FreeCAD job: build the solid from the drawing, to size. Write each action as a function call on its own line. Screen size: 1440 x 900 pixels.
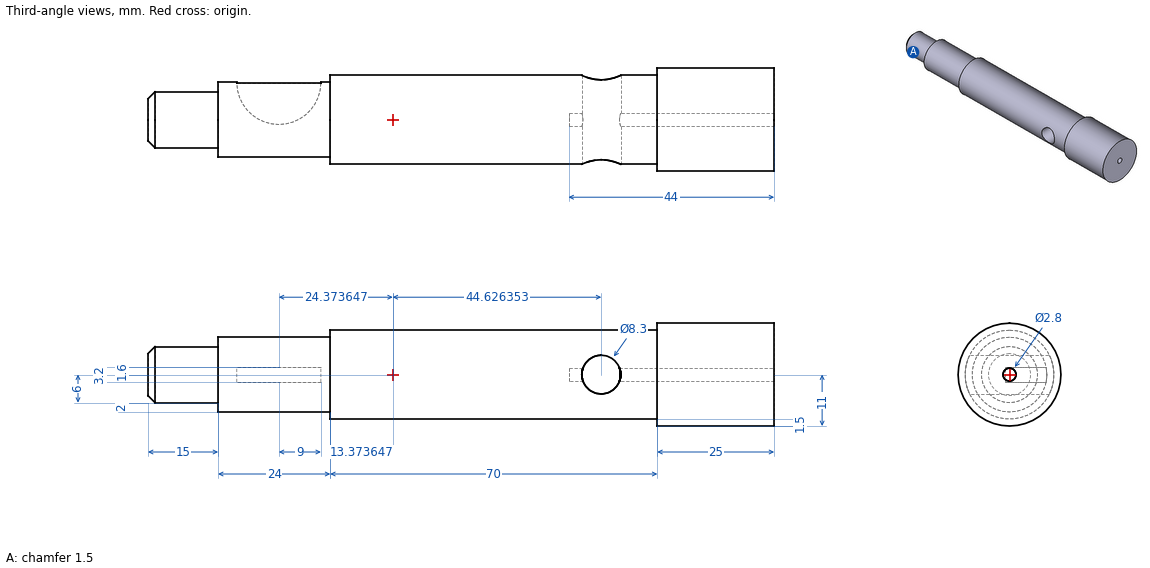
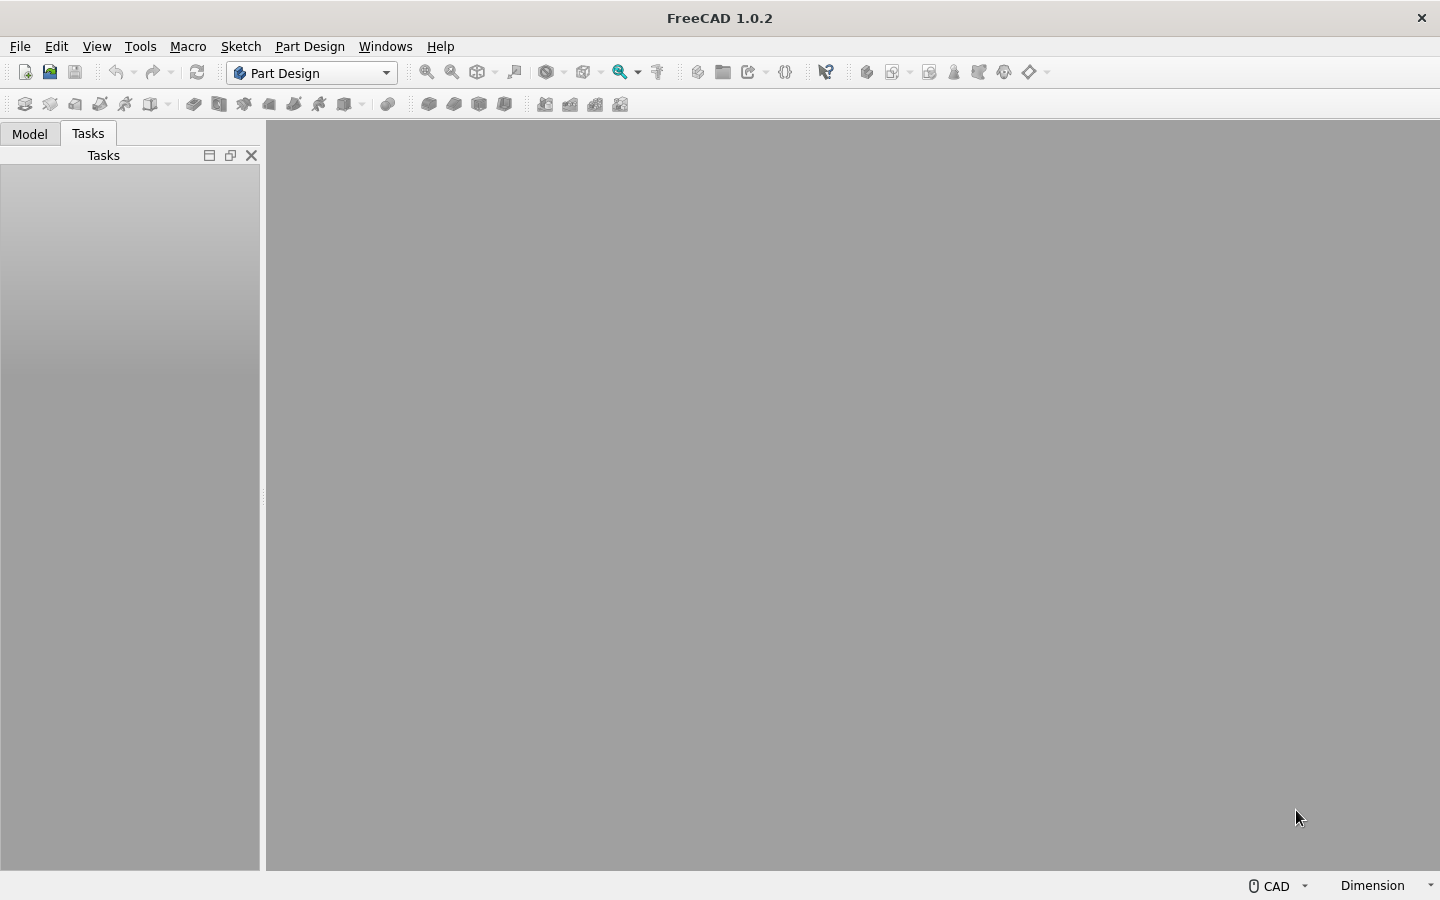
click(25, 72)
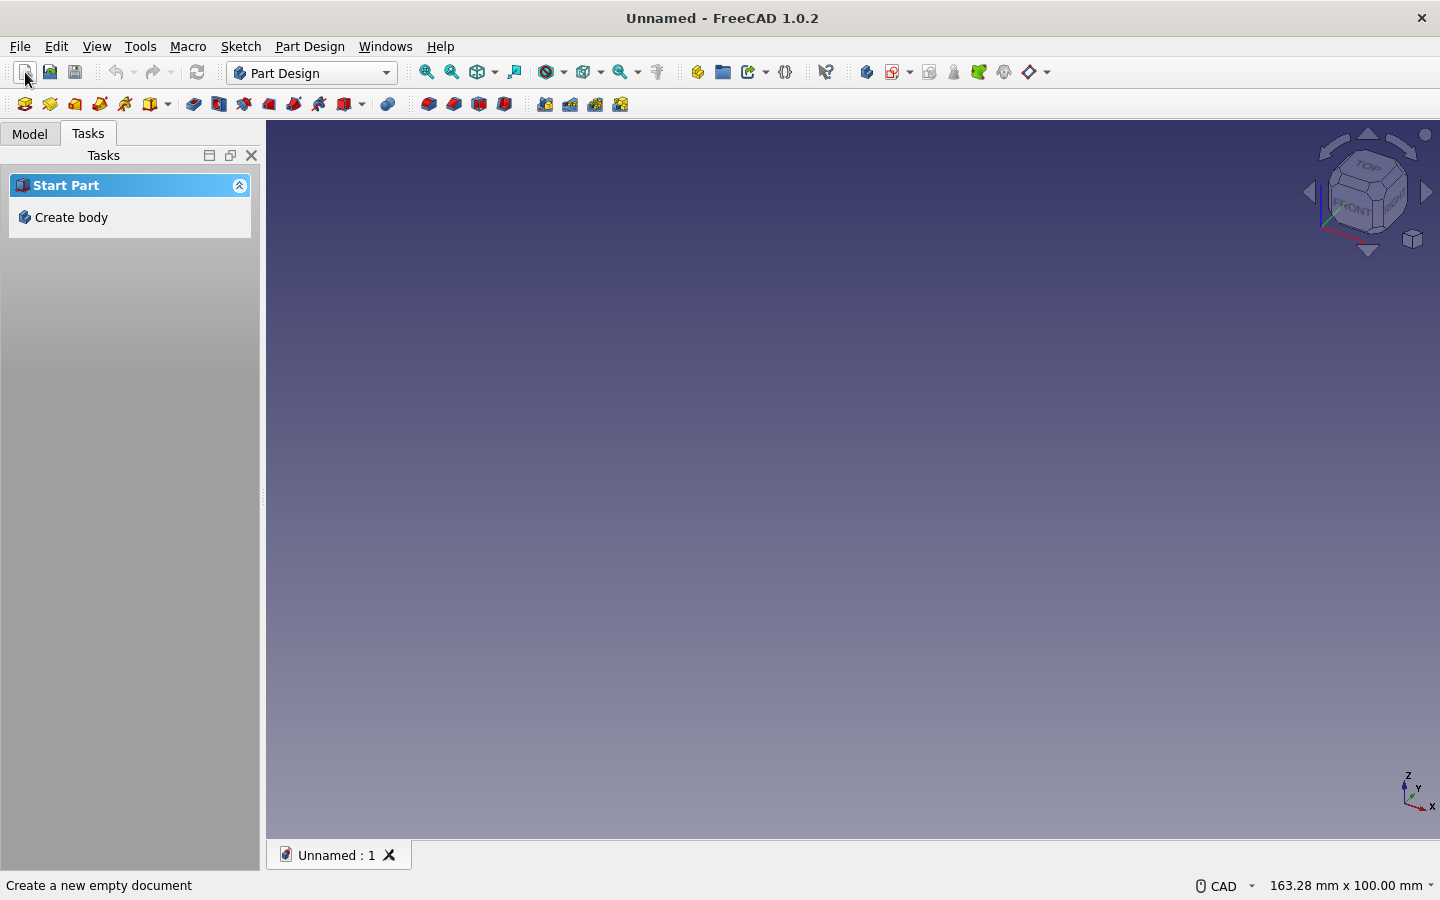
click(892, 72)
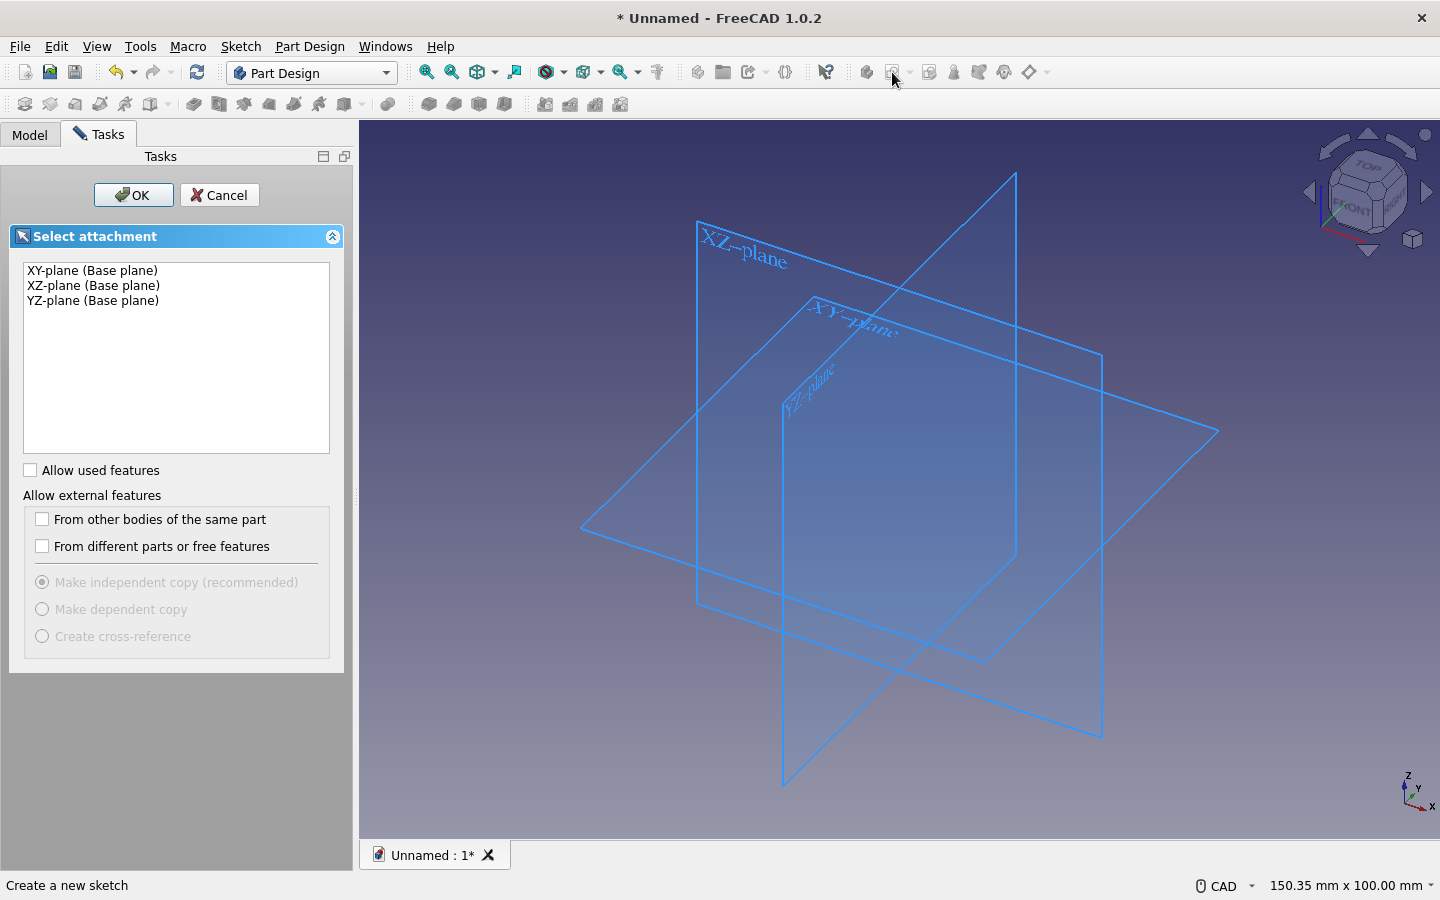
click(84, 286)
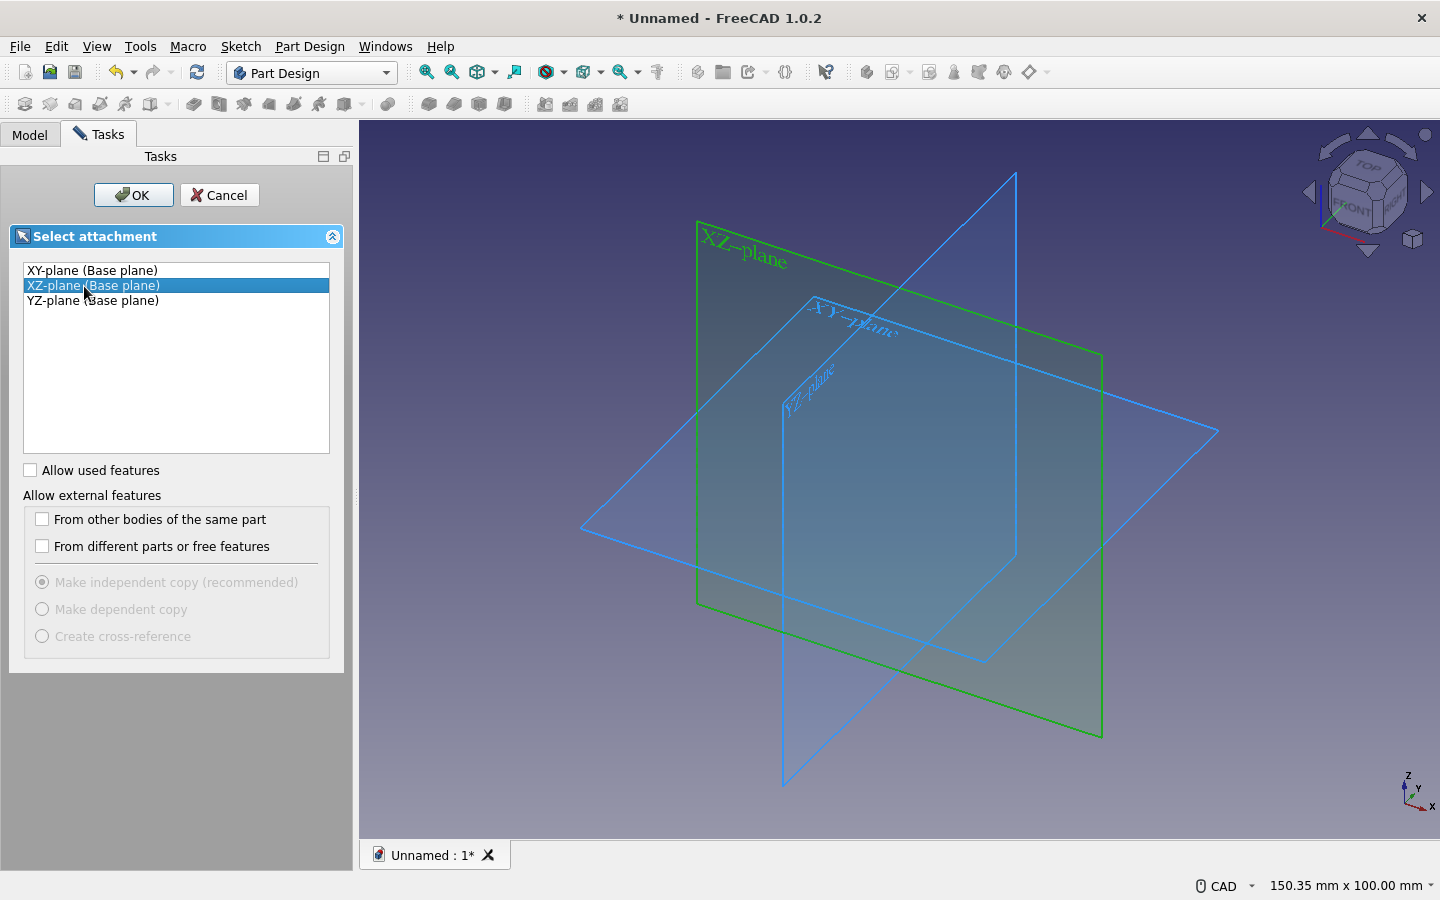
click(134, 195)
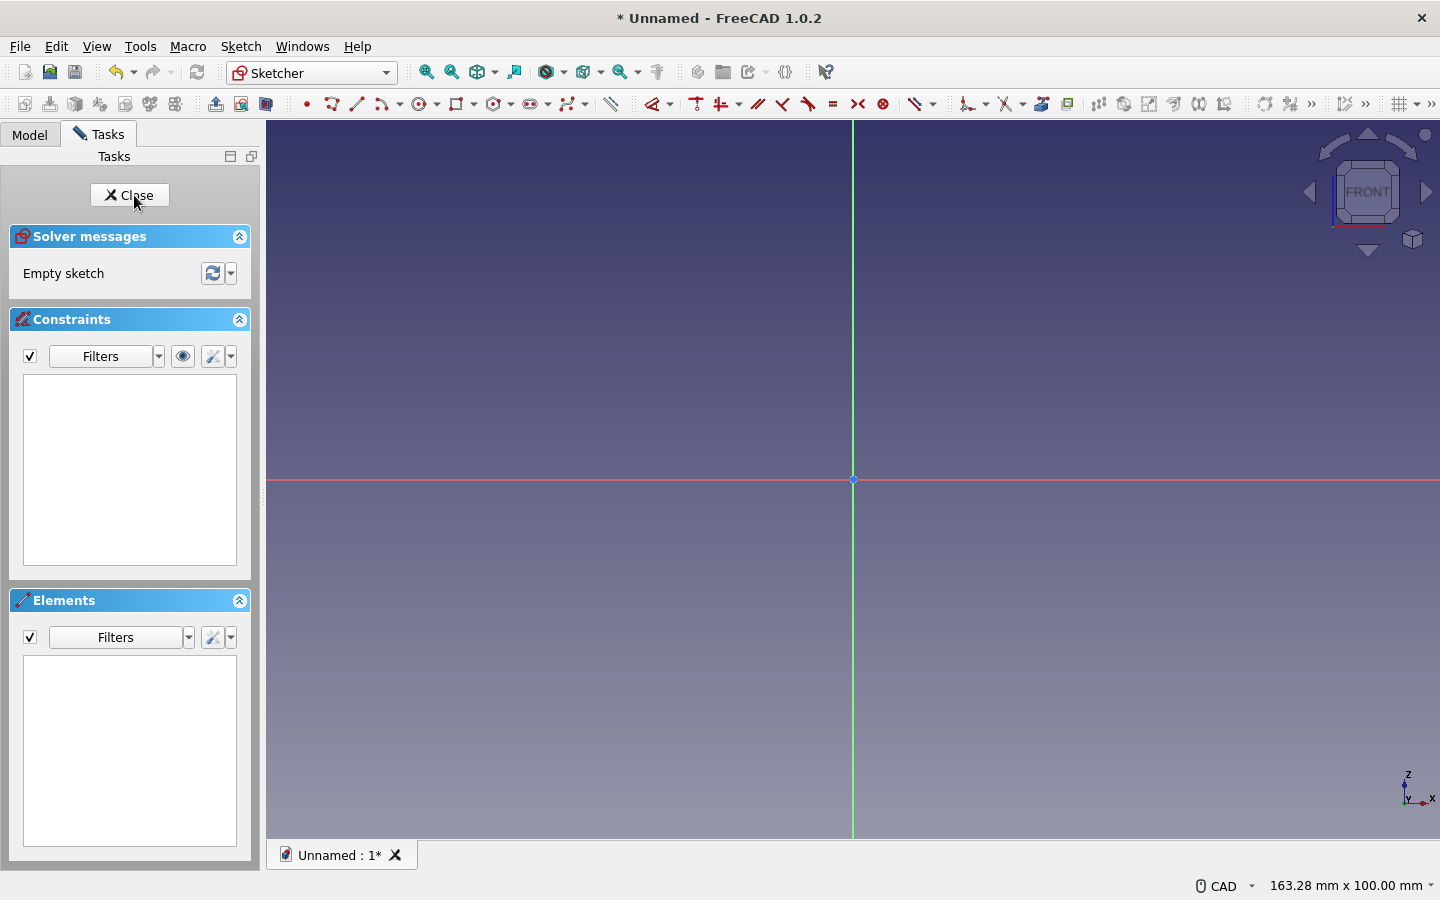
scroll(431, 399, down, 2)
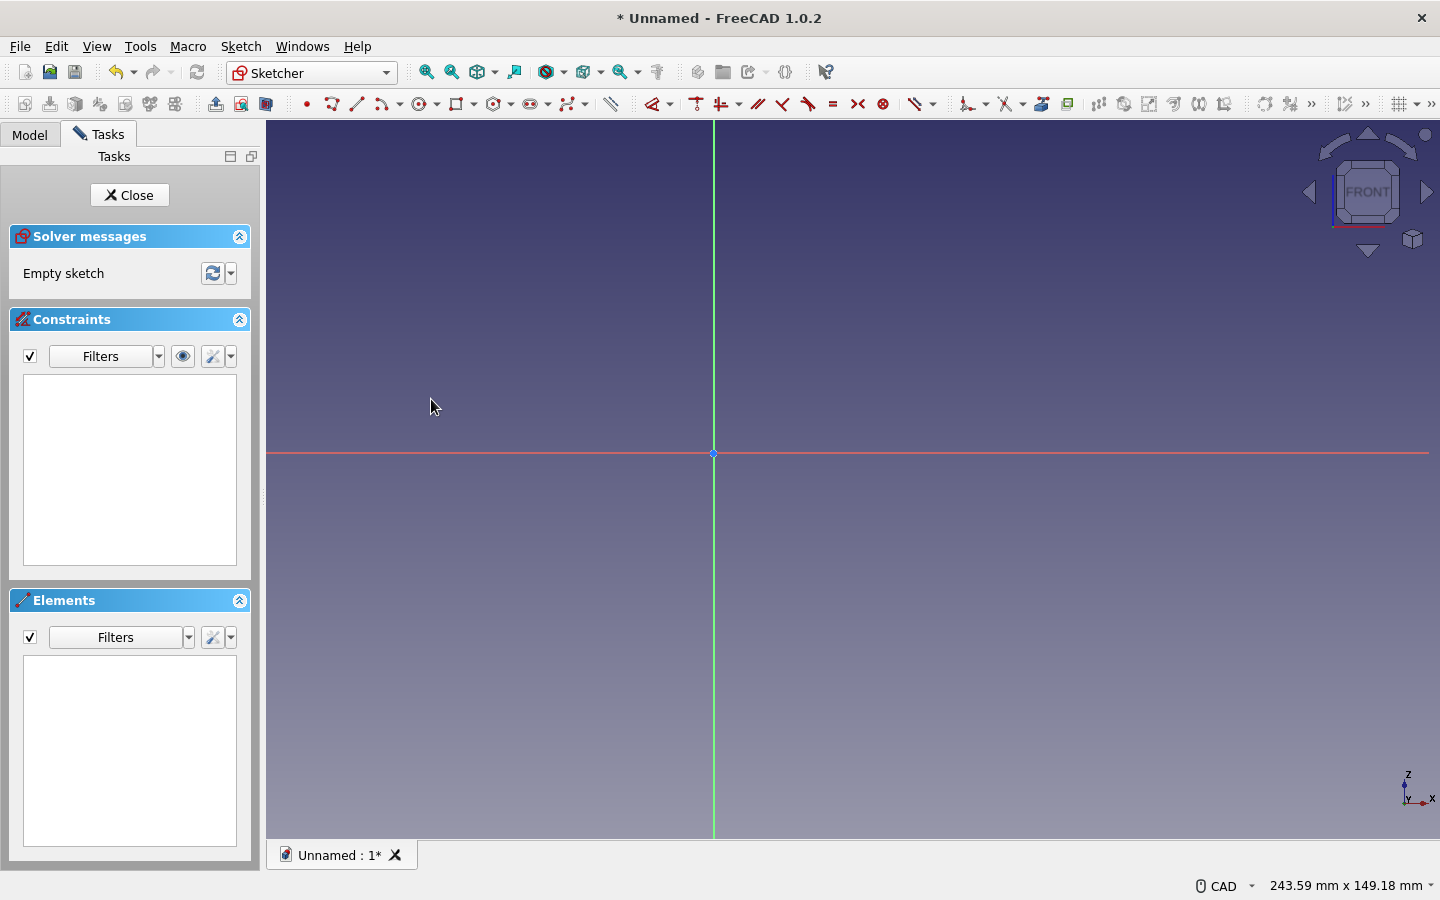
click(332, 104)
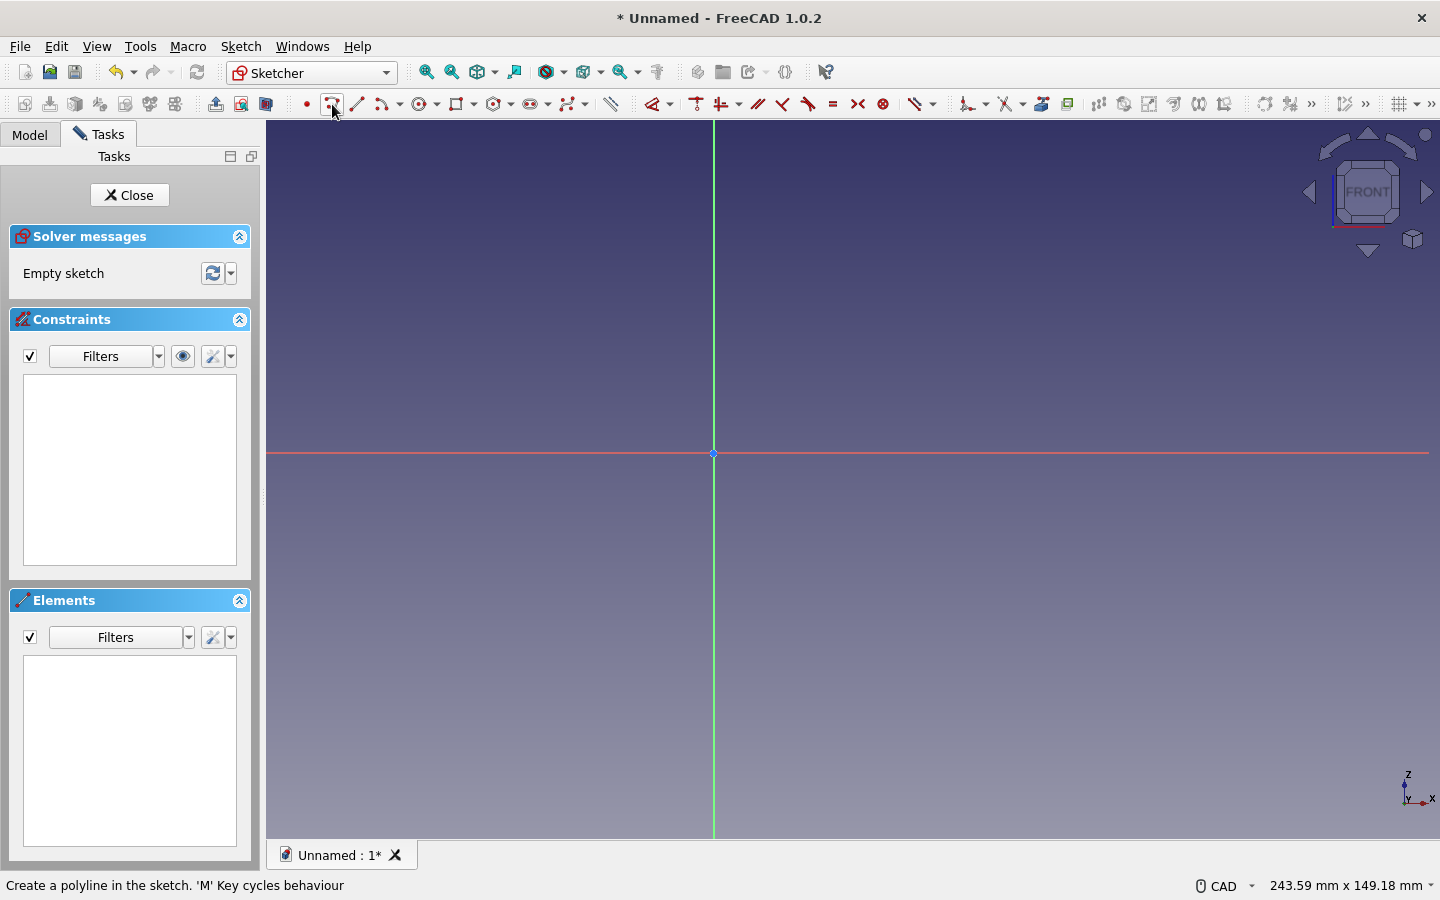
click(649, 492)
click(534, 492)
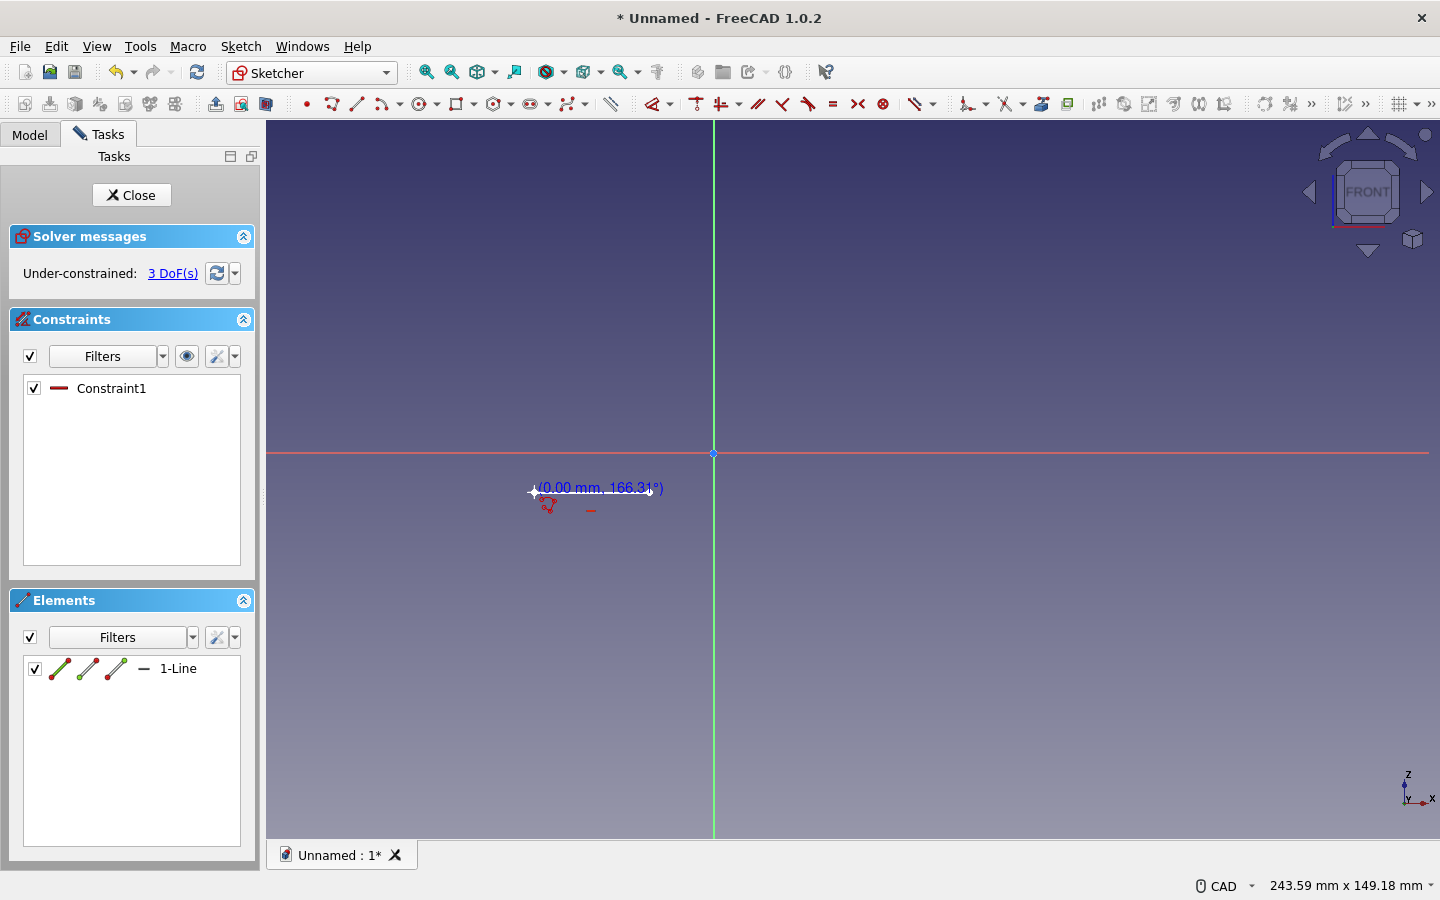
scroll(534, 482, up, 3)